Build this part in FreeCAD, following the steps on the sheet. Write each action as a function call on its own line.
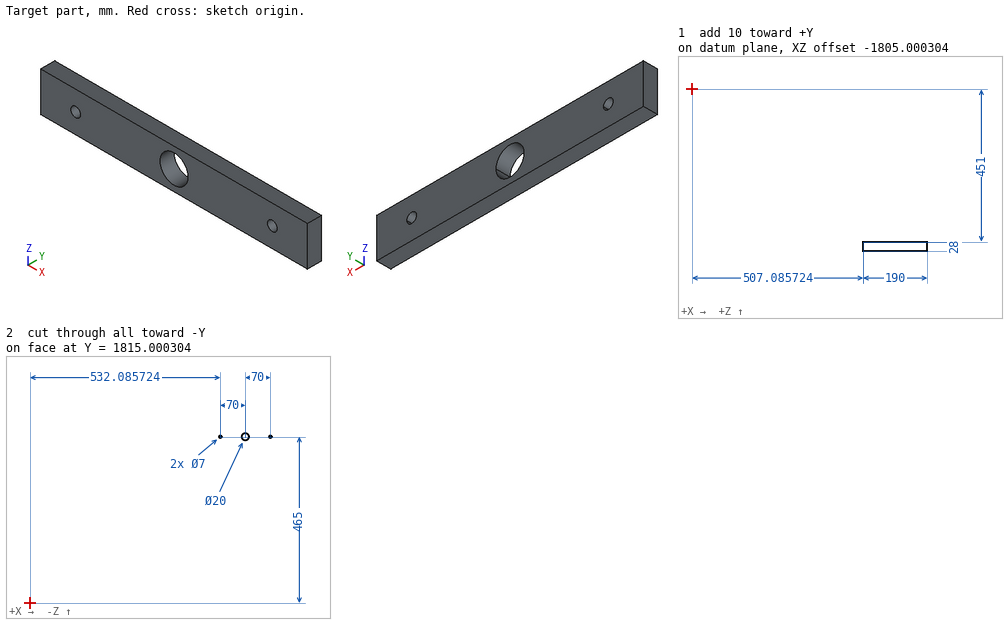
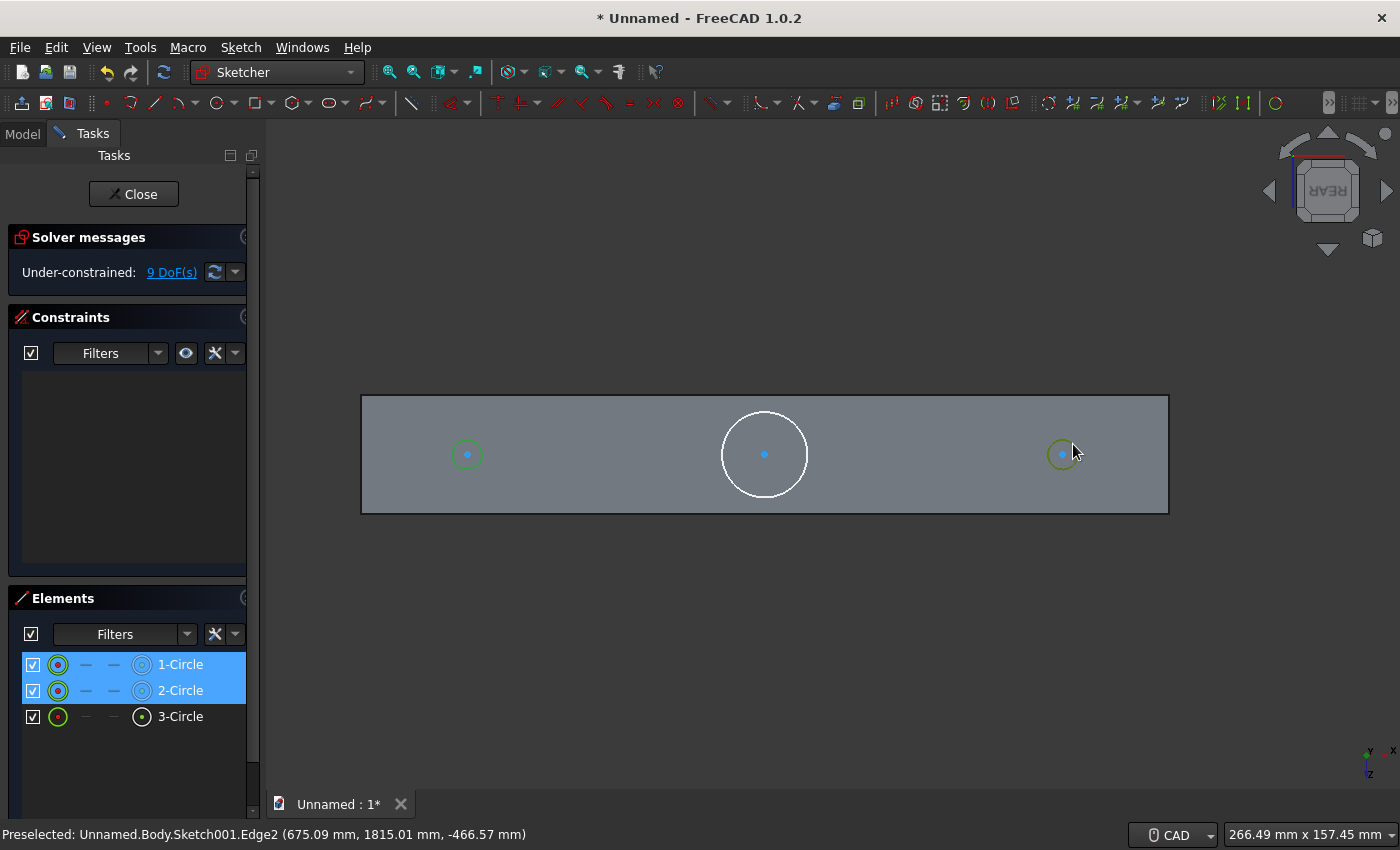
click(630, 104)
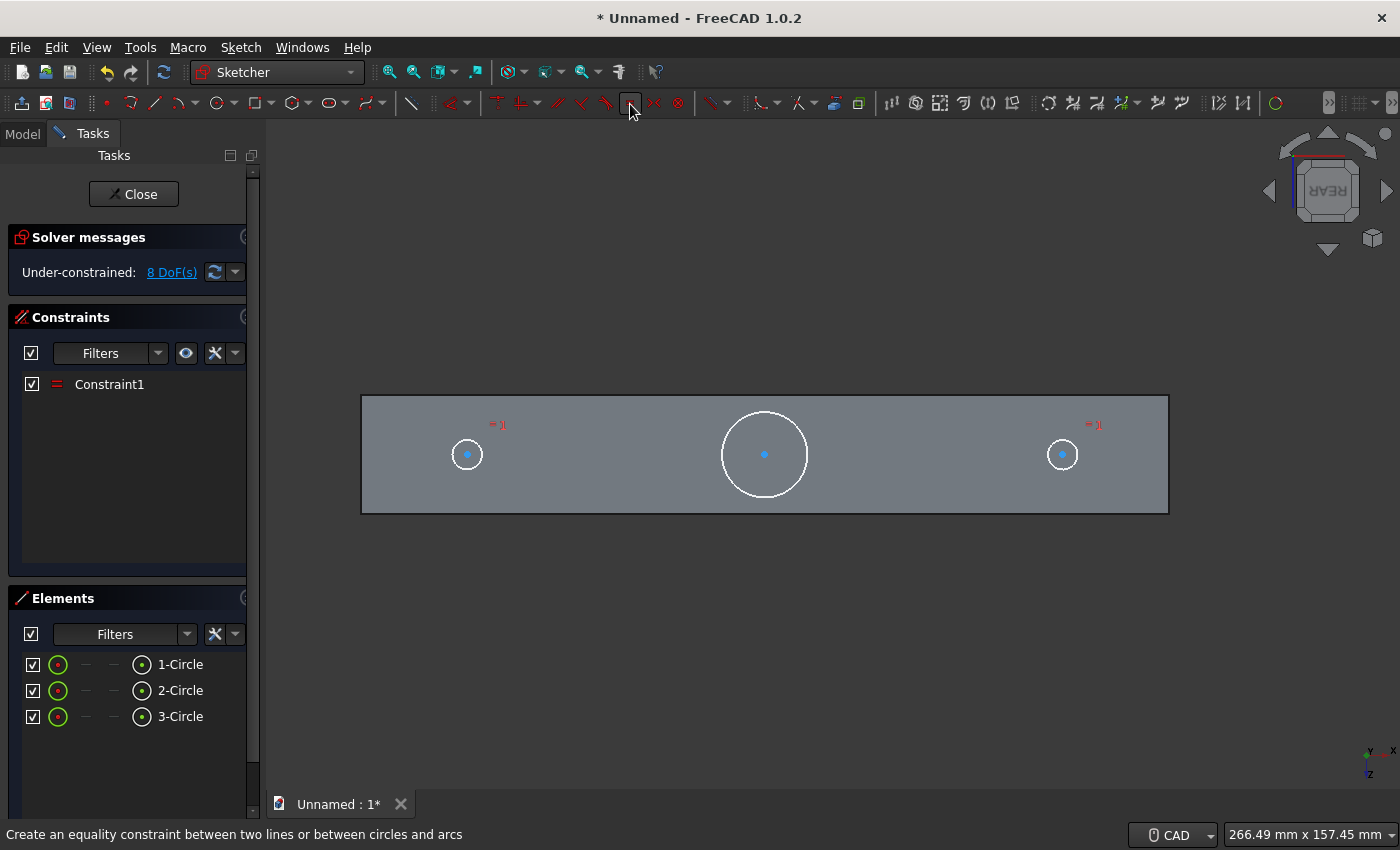
click(467, 455)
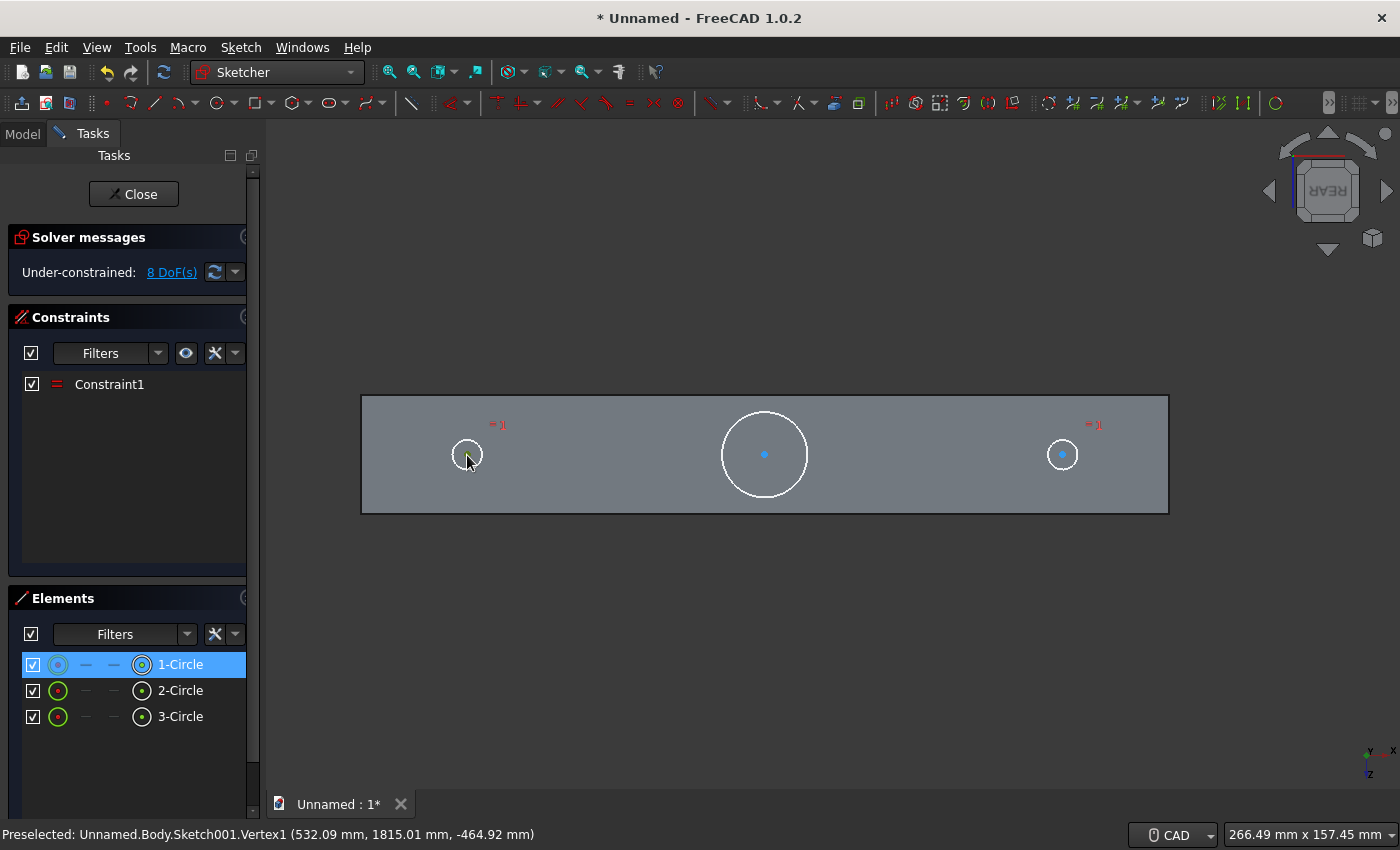
click(1063, 455)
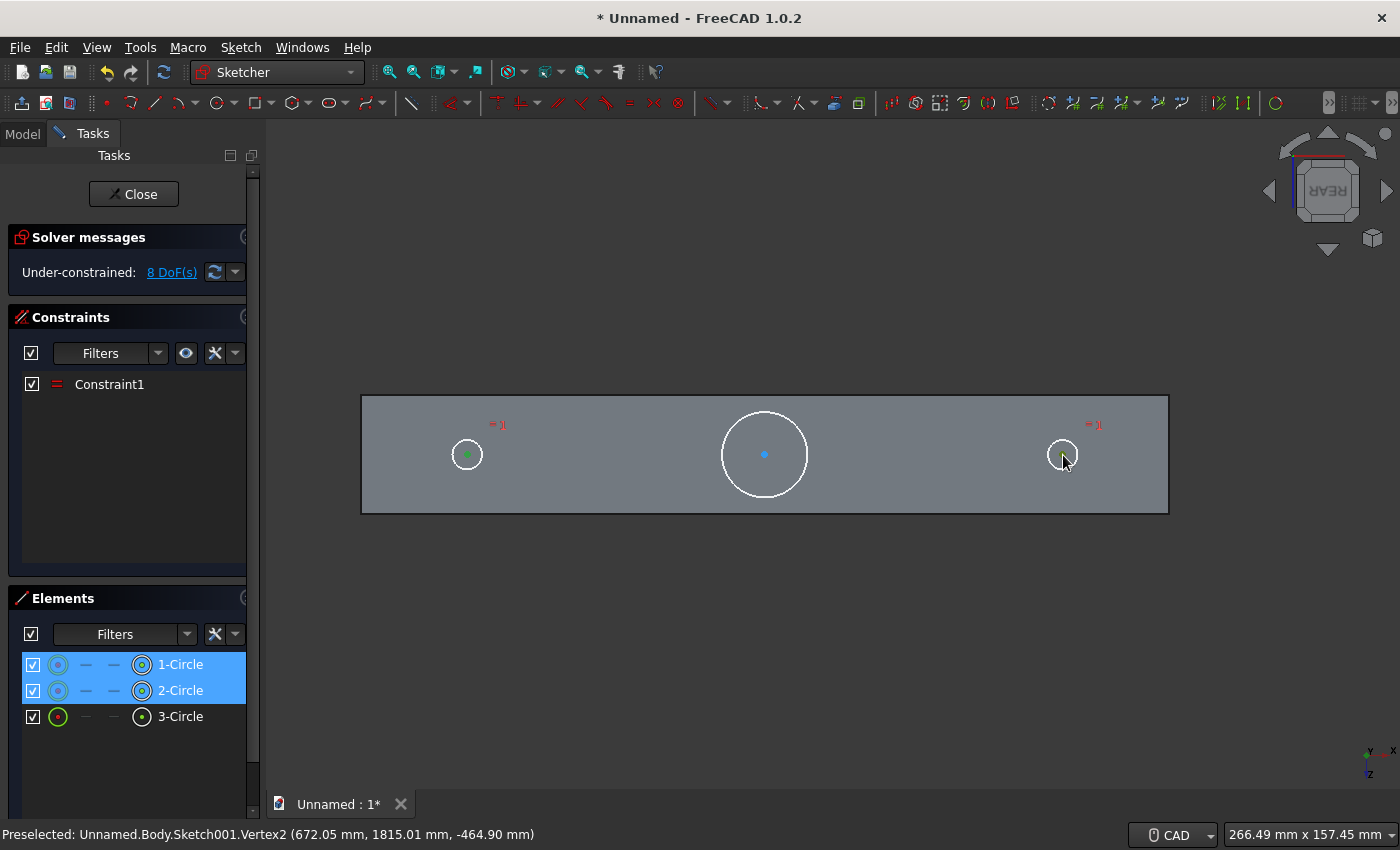
key(h)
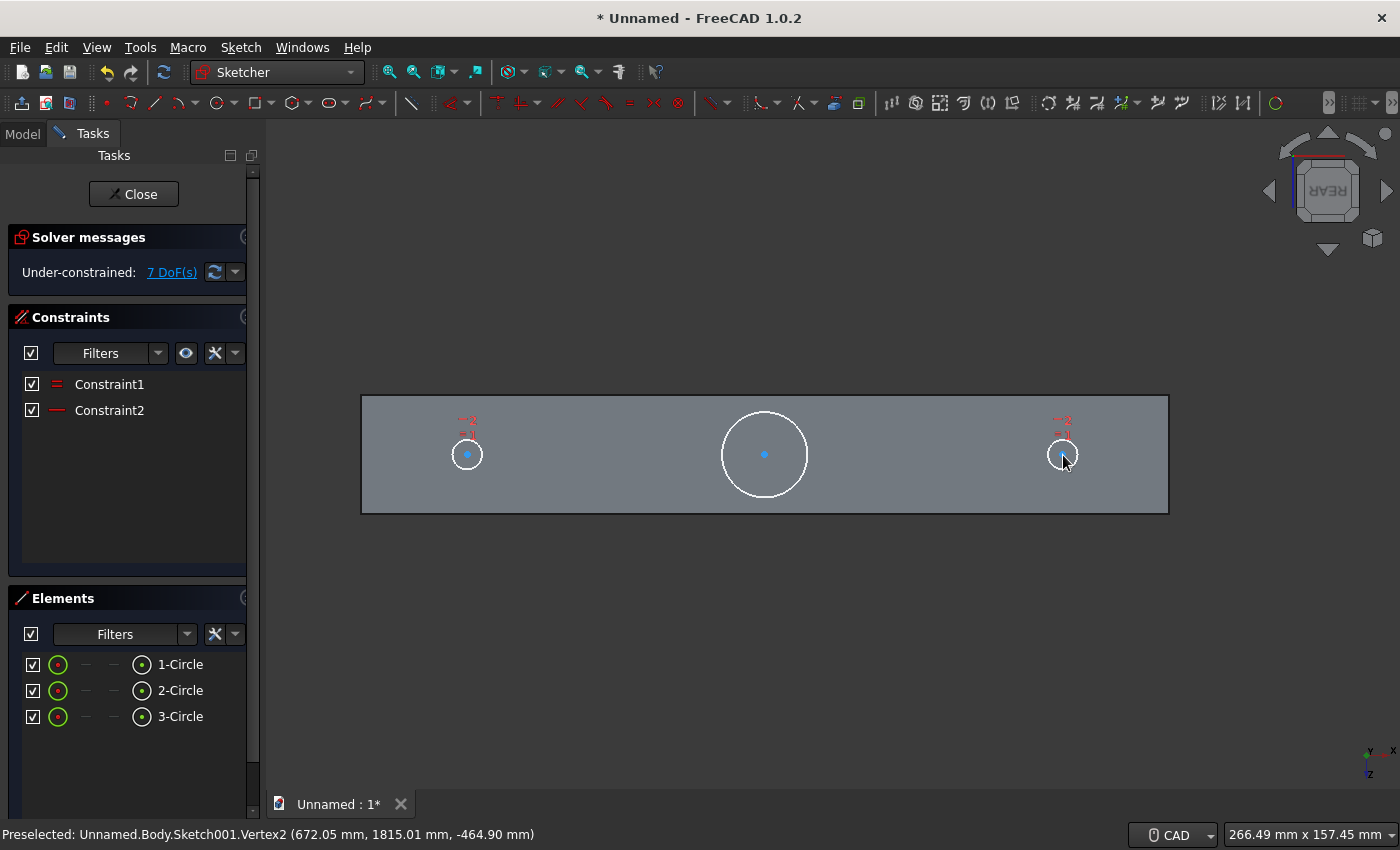
click(467, 455)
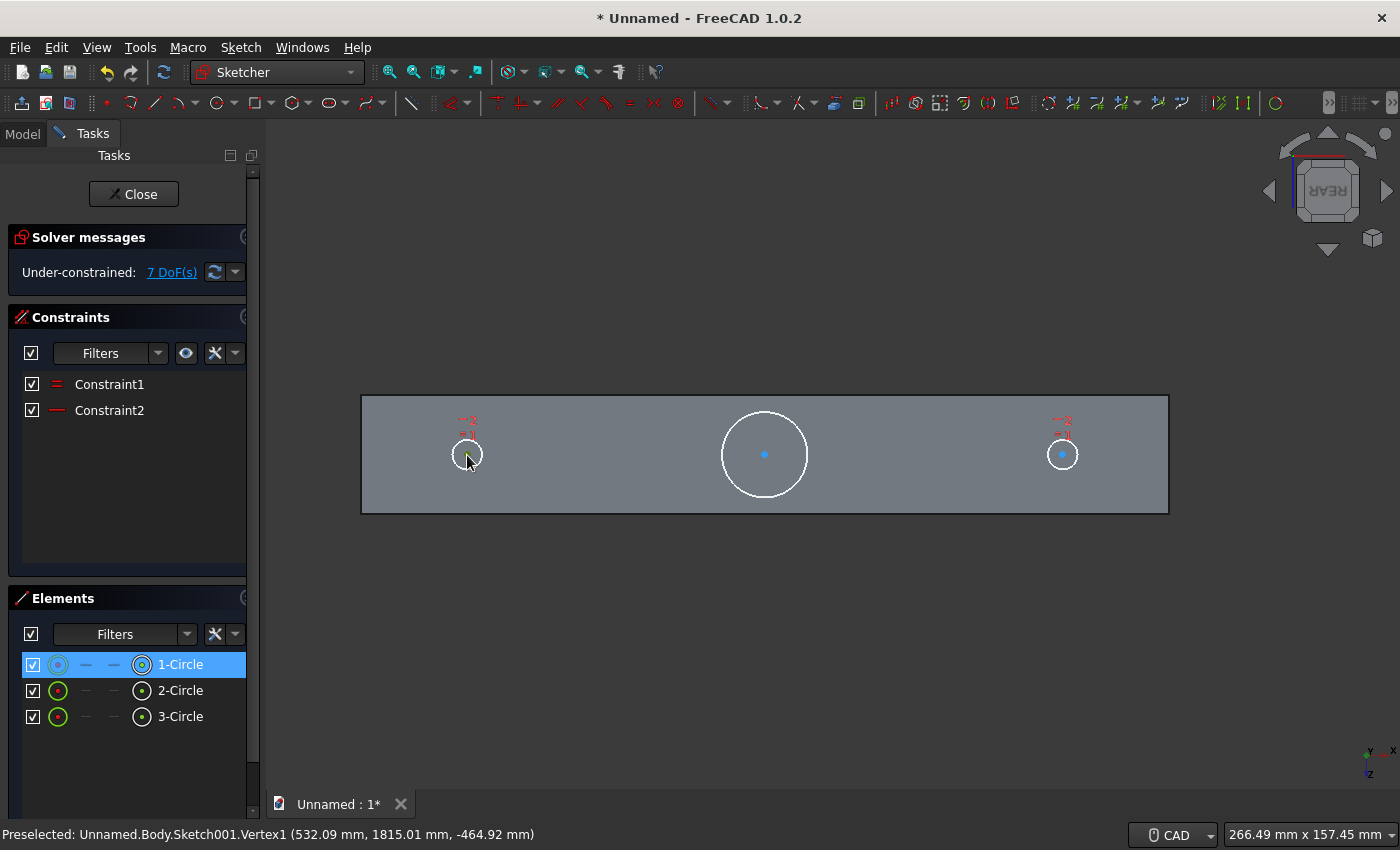
click(765, 455)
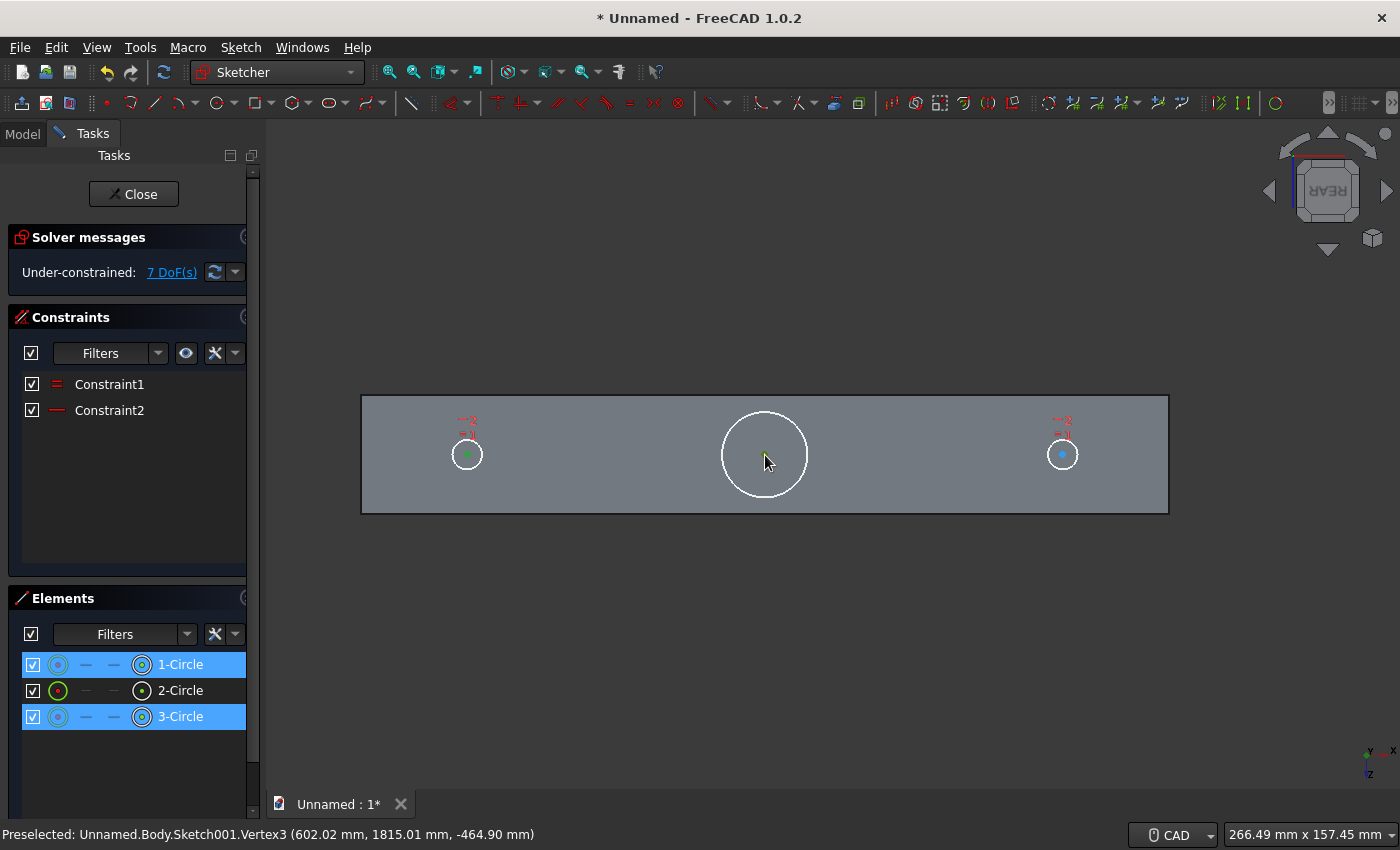
key(h)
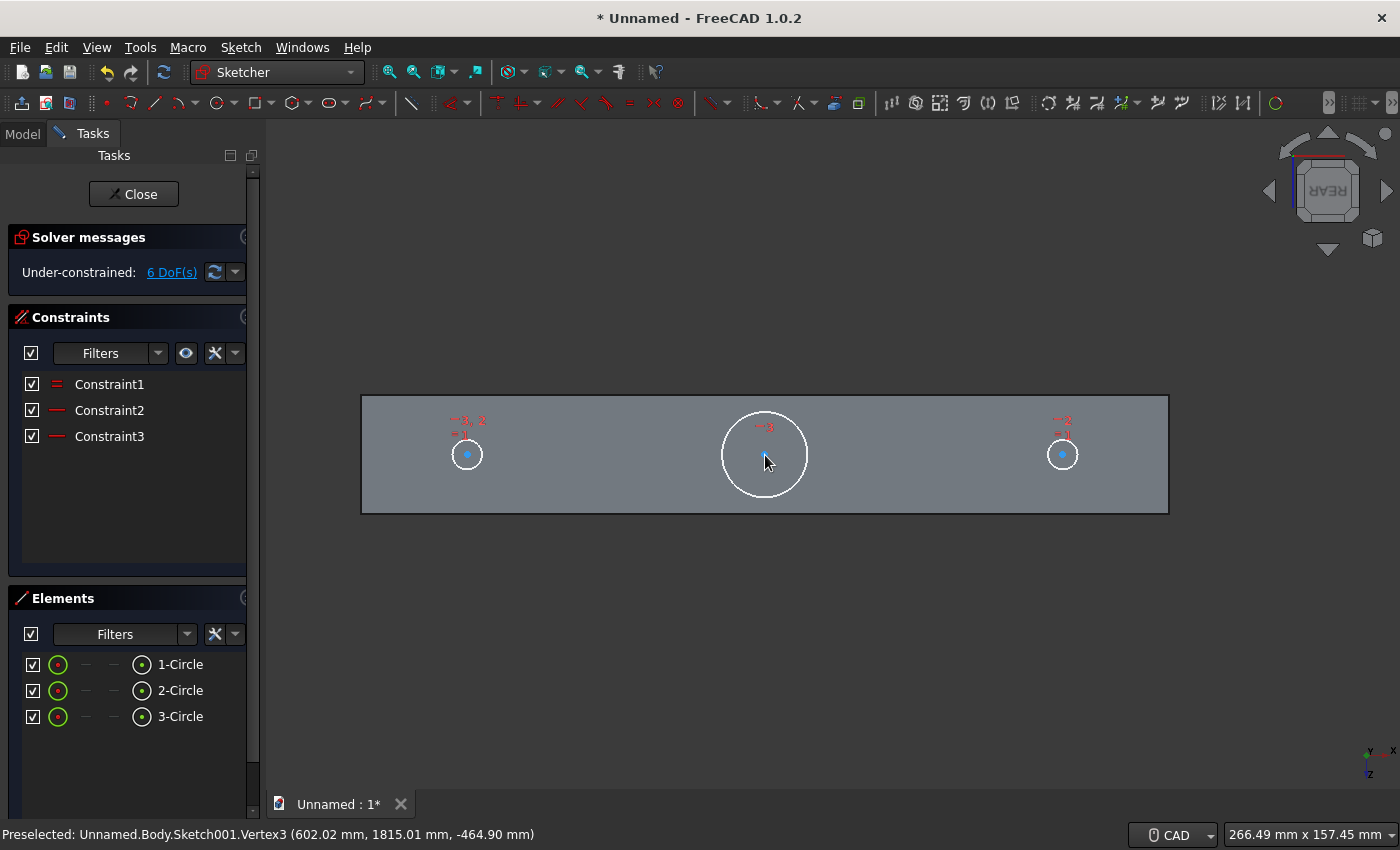
click(450, 104)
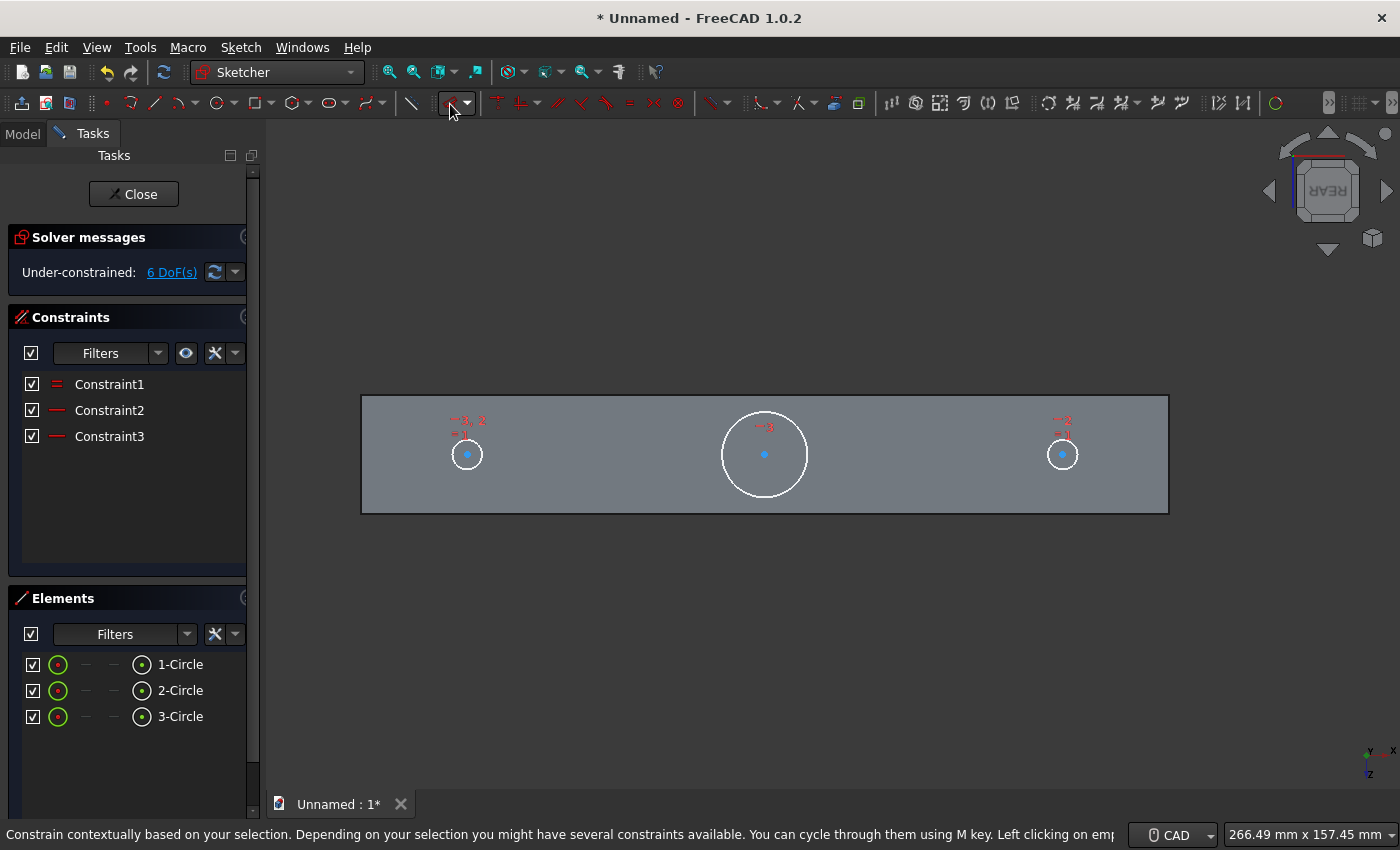
scroll(478, 444, up, 2)